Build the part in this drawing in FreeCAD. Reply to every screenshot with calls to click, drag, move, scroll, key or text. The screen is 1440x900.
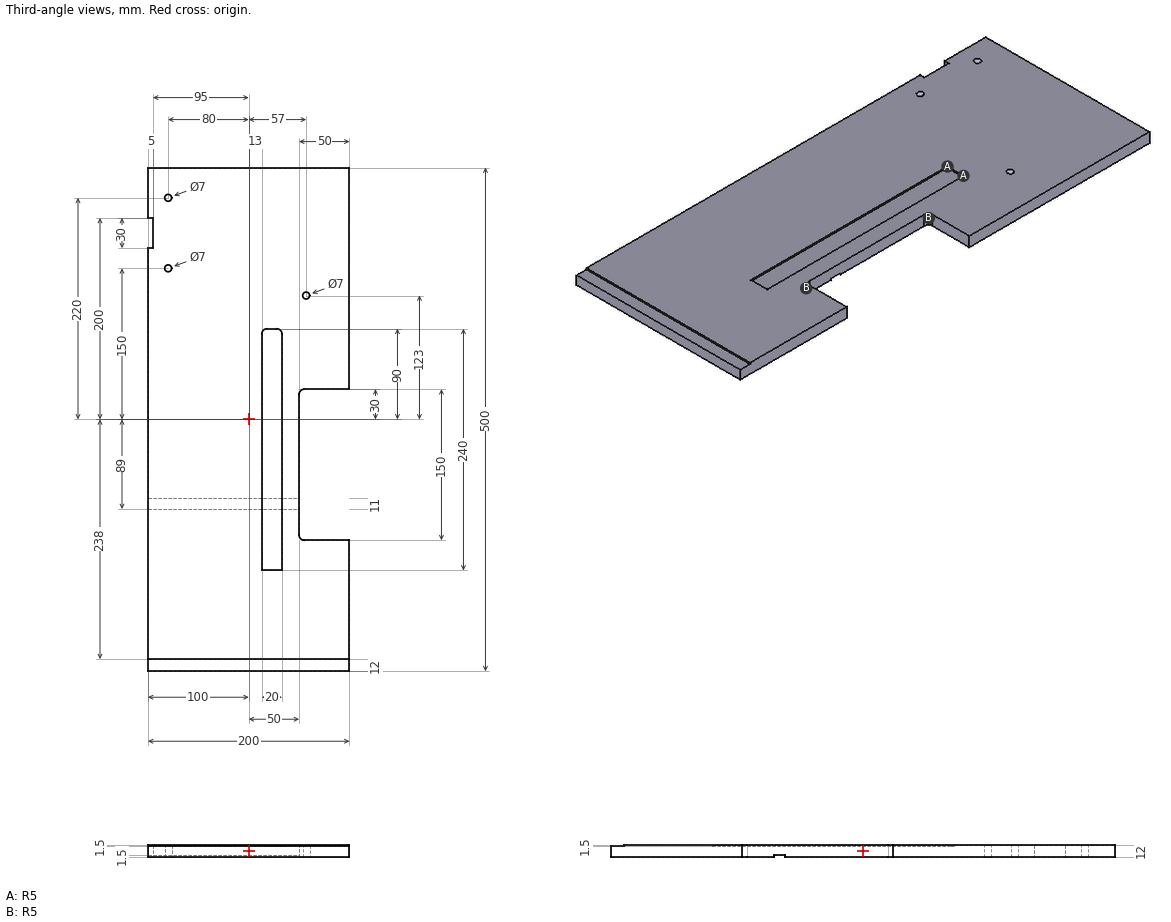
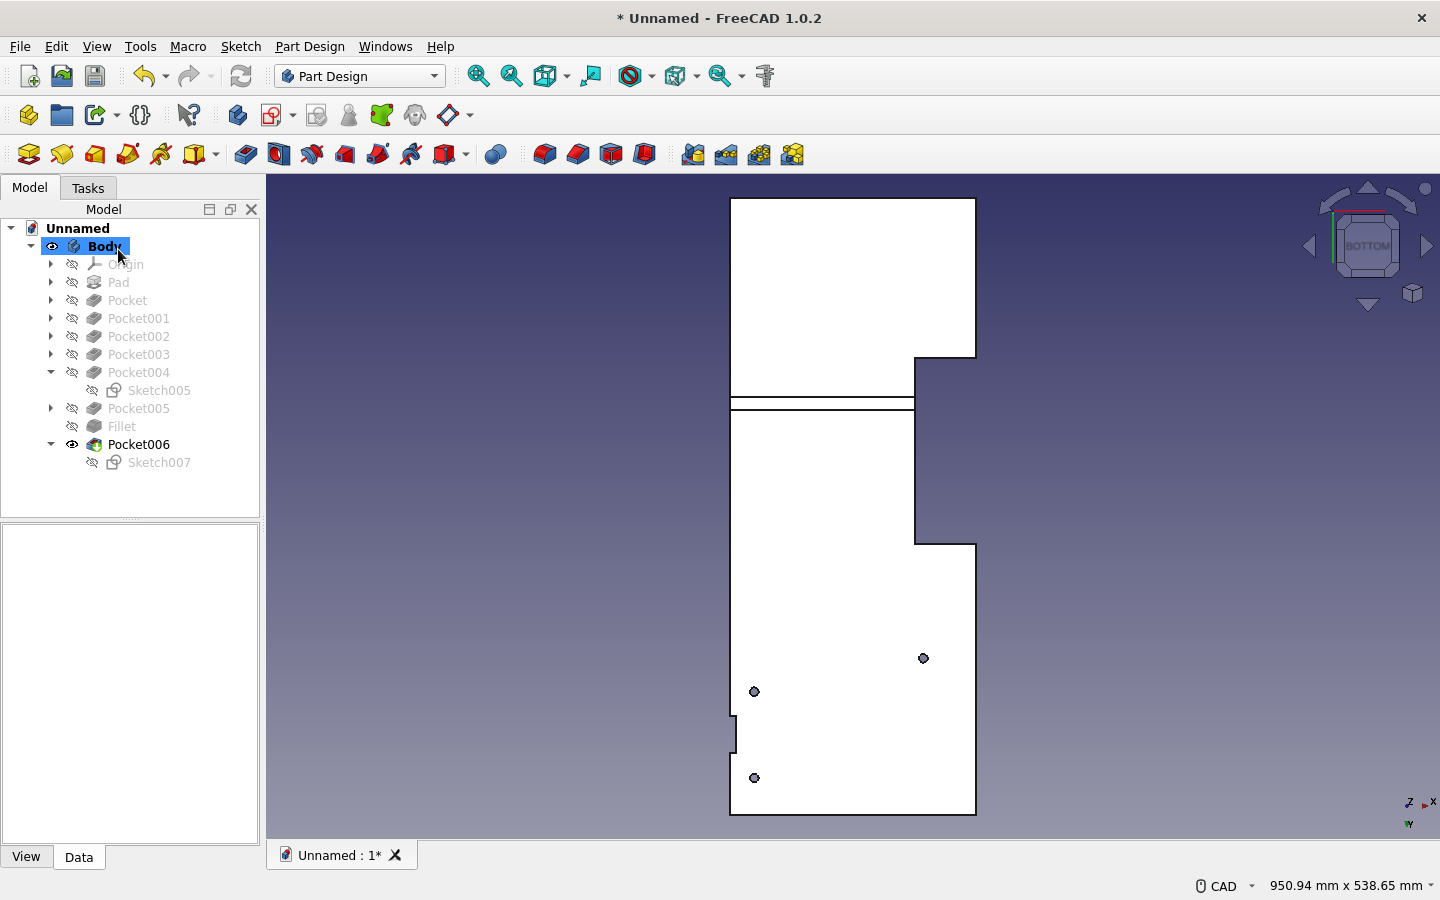
scroll(915, 543, up, 5)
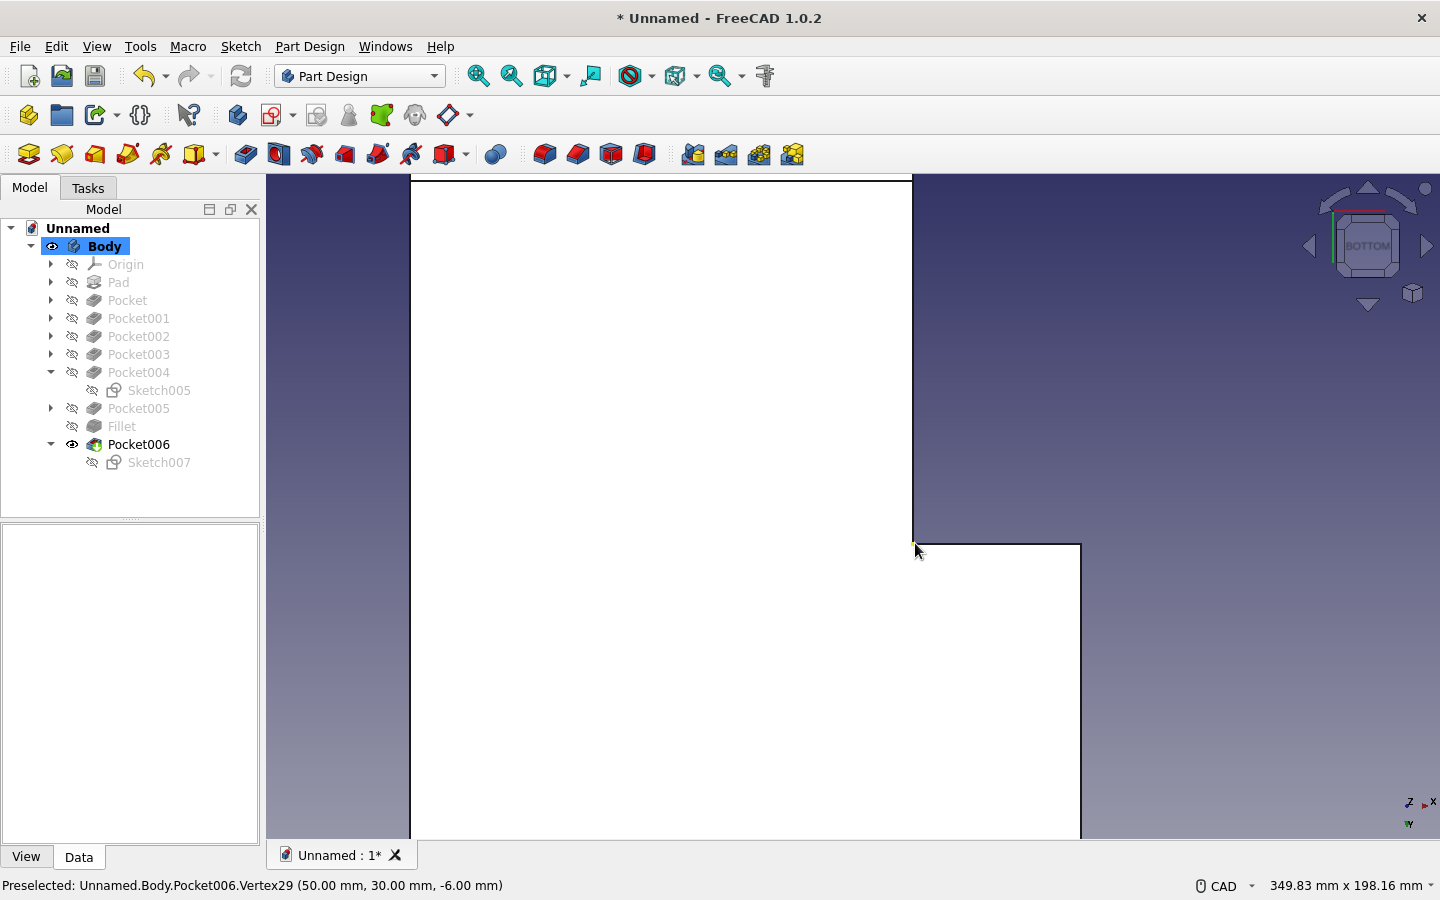
click(479, 76)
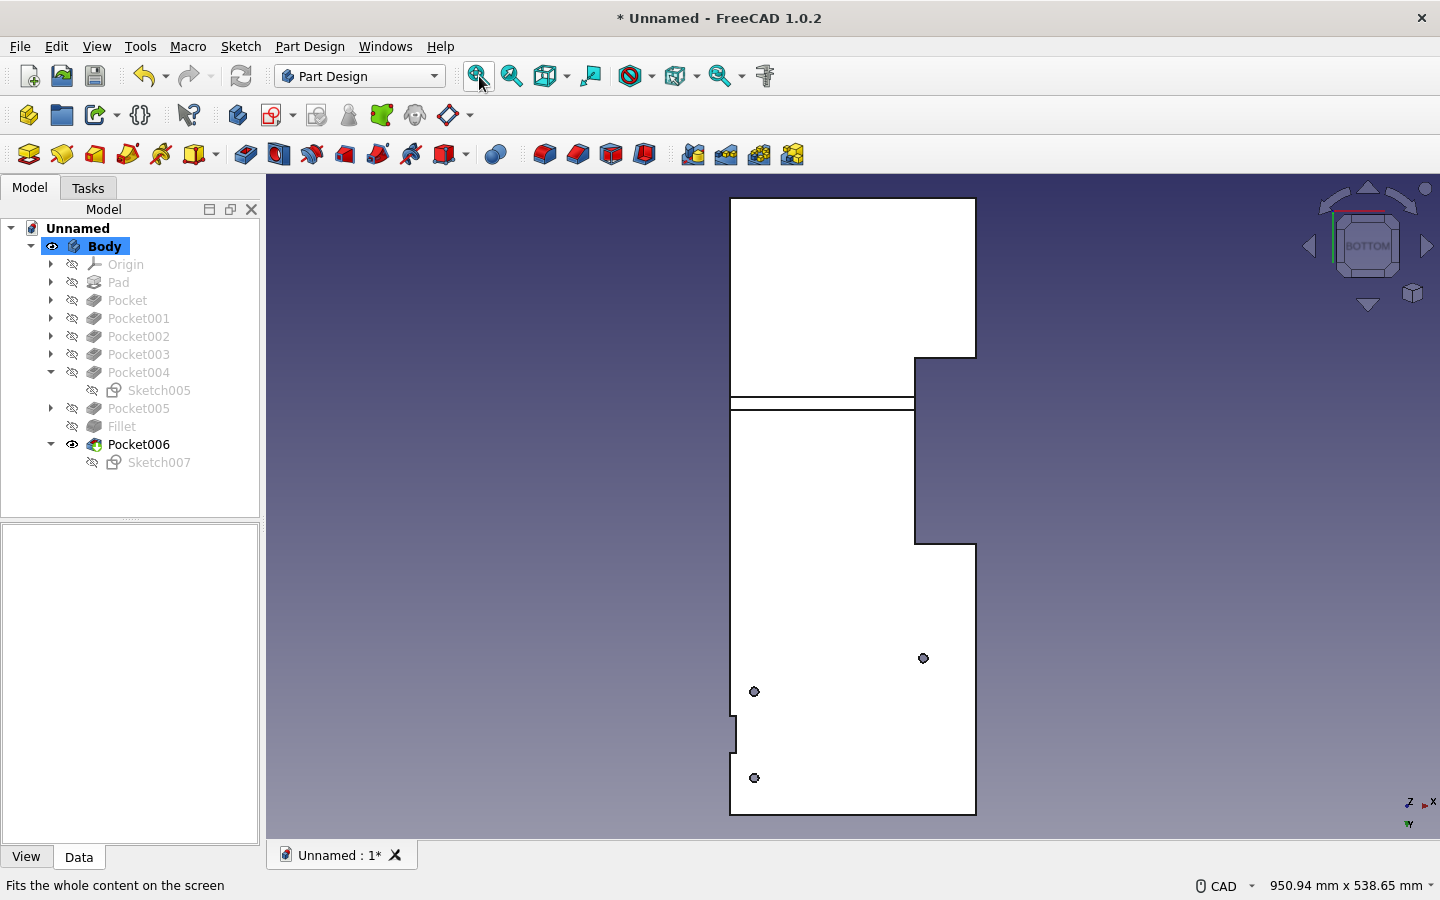
key(0)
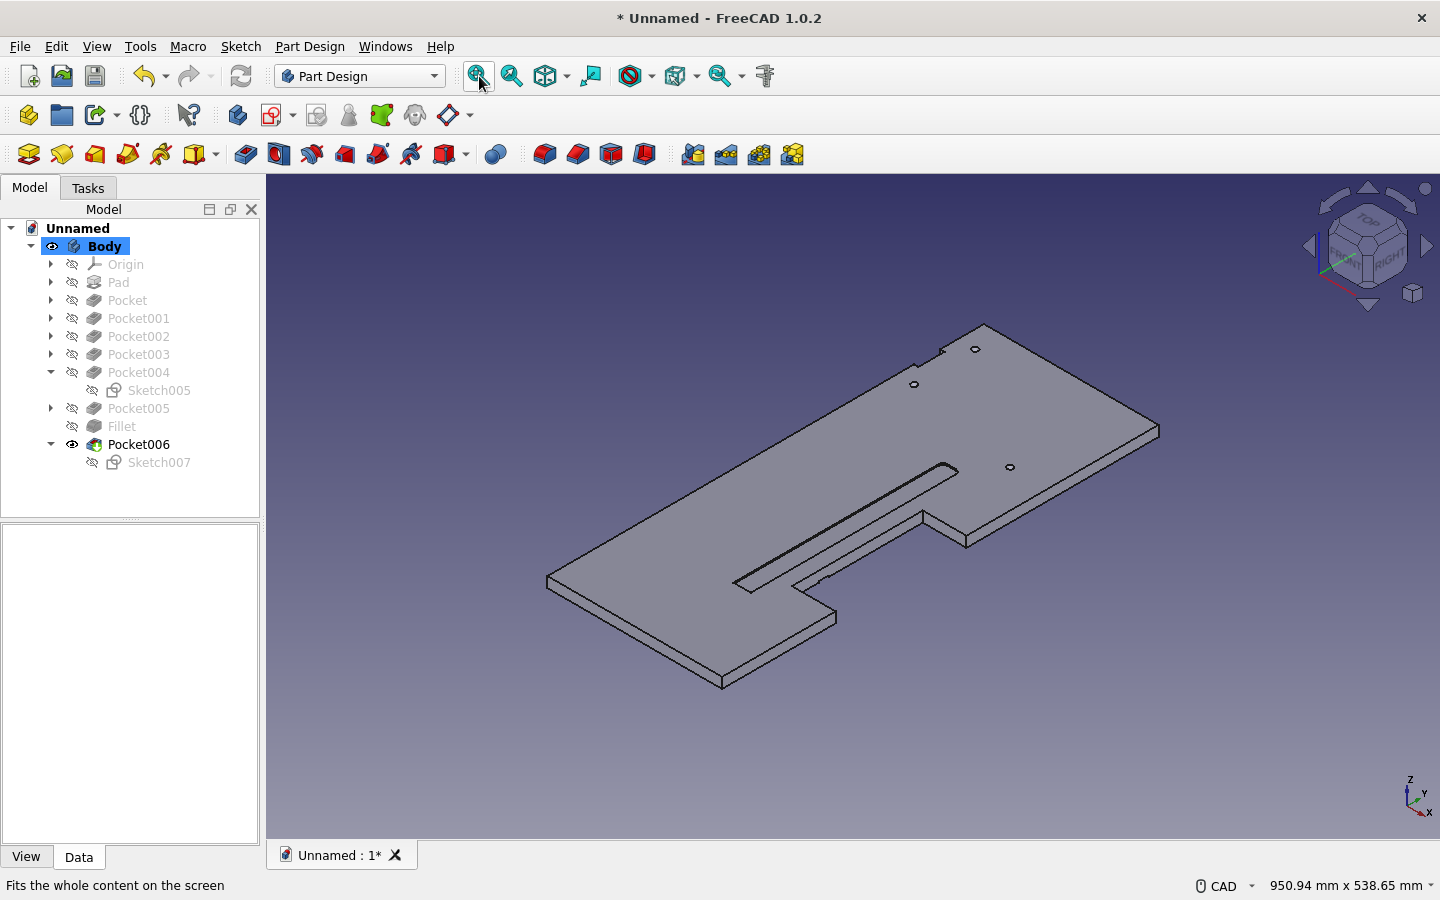
scroll(923, 516, up, 5)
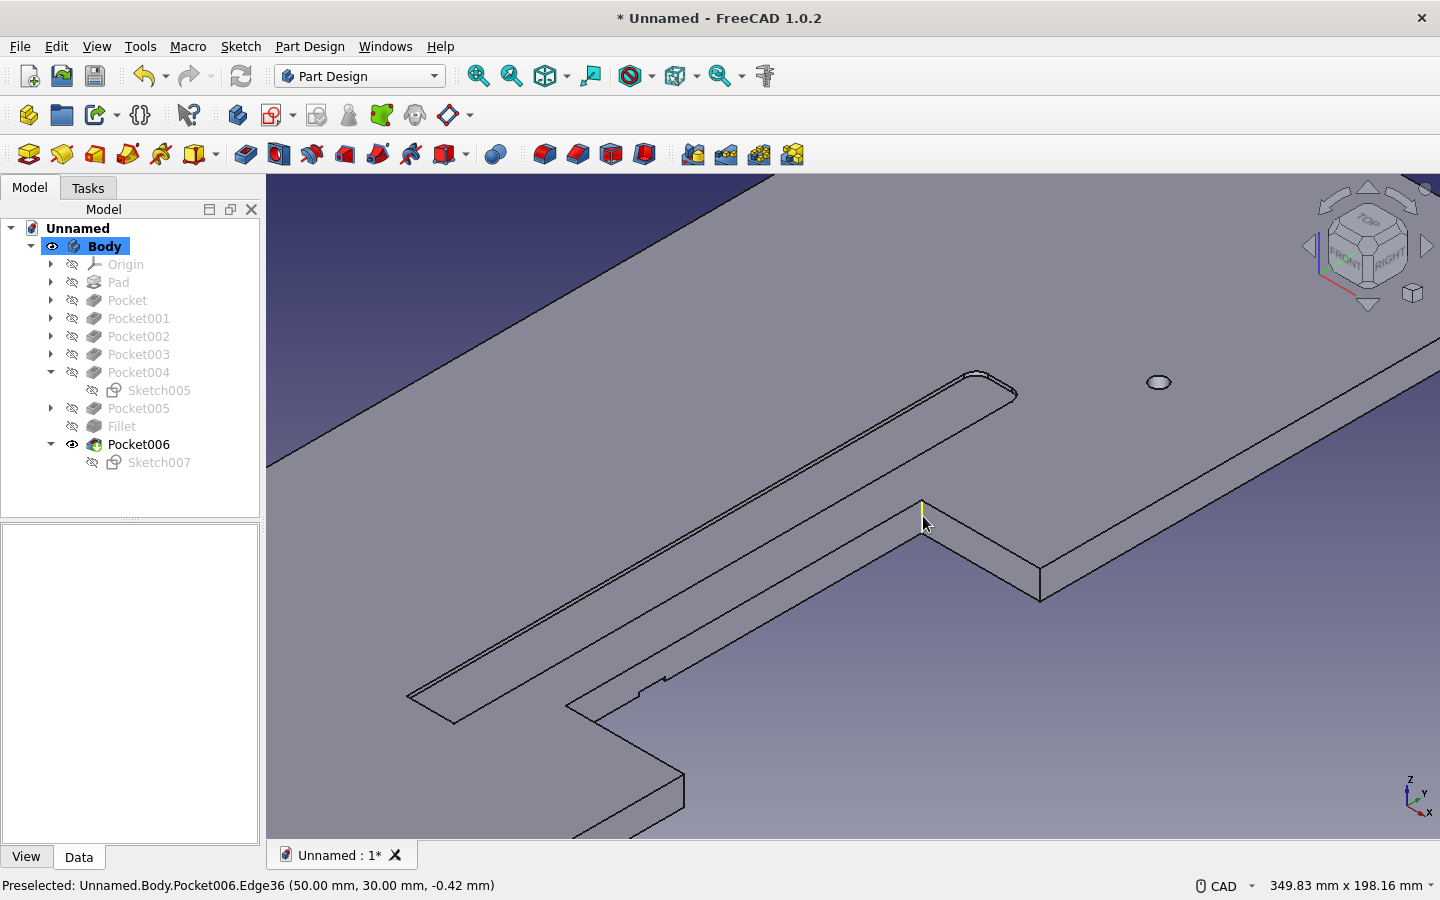
click(479, 76)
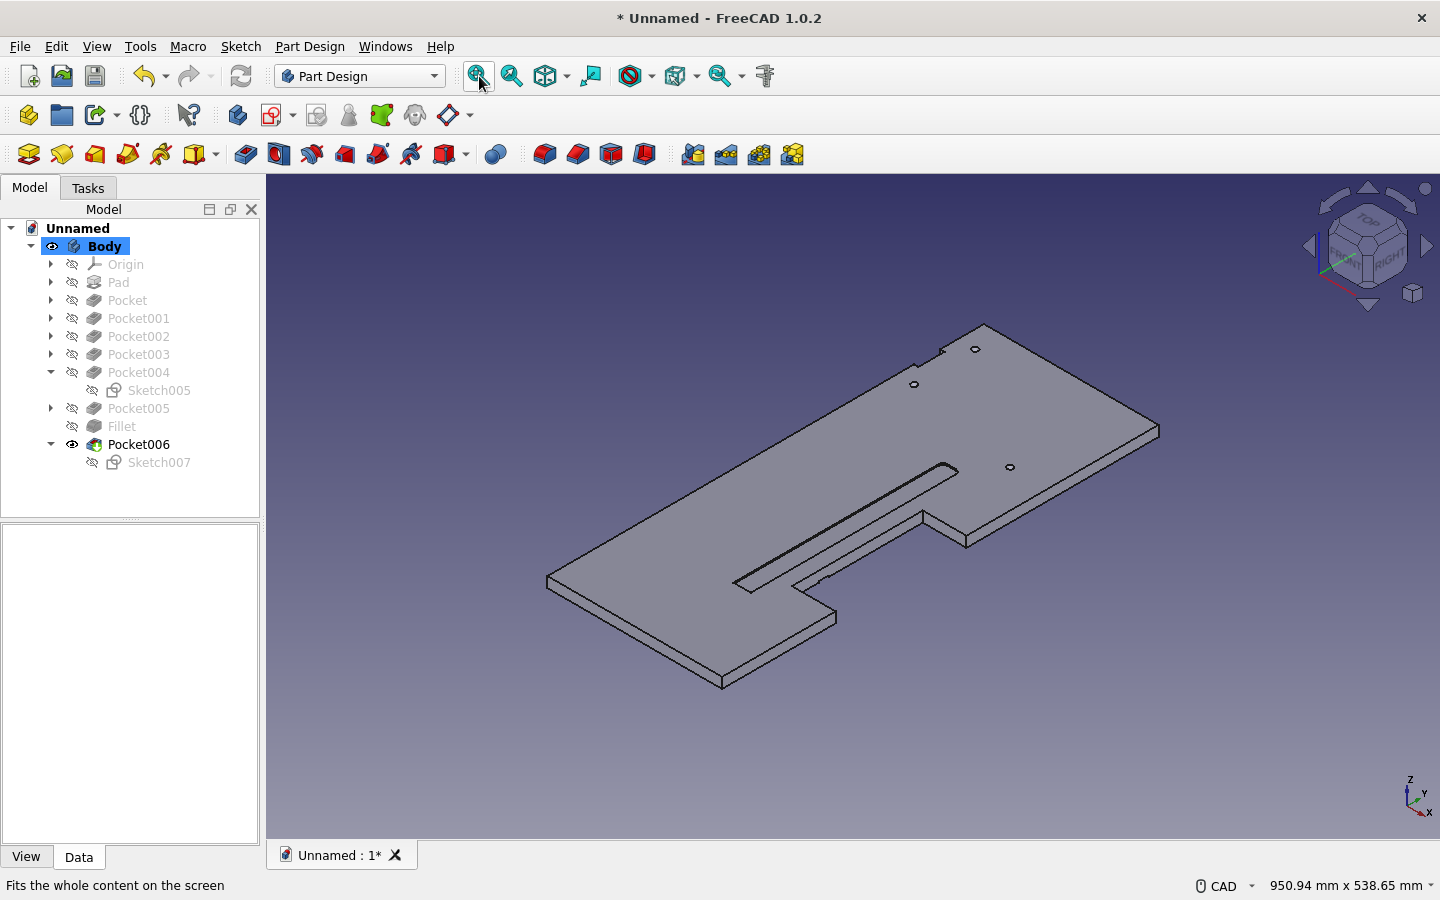
key(2)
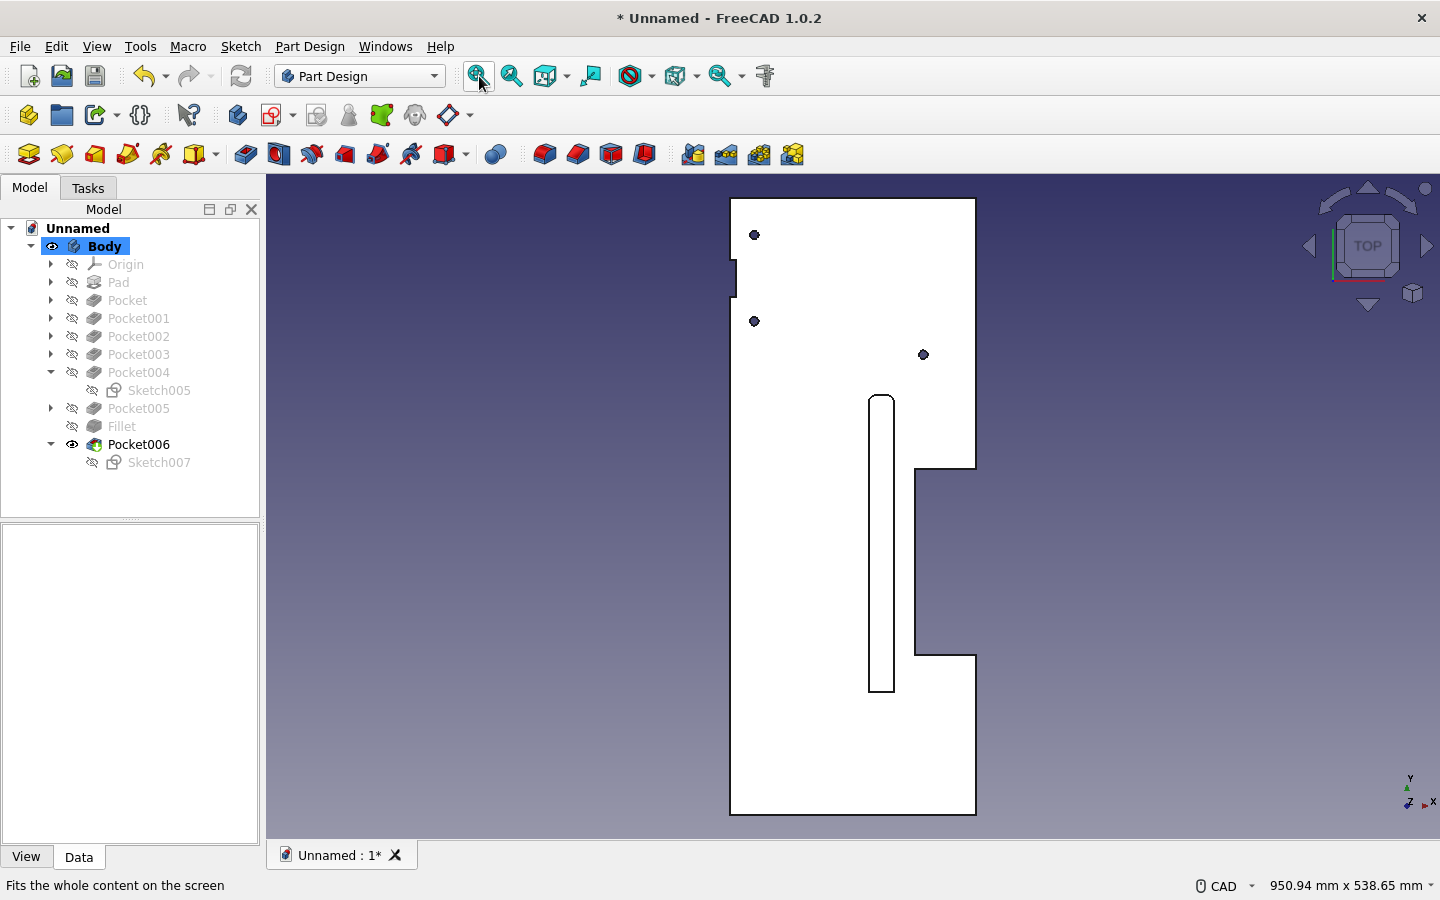
scroll(915, 468, up, 5)